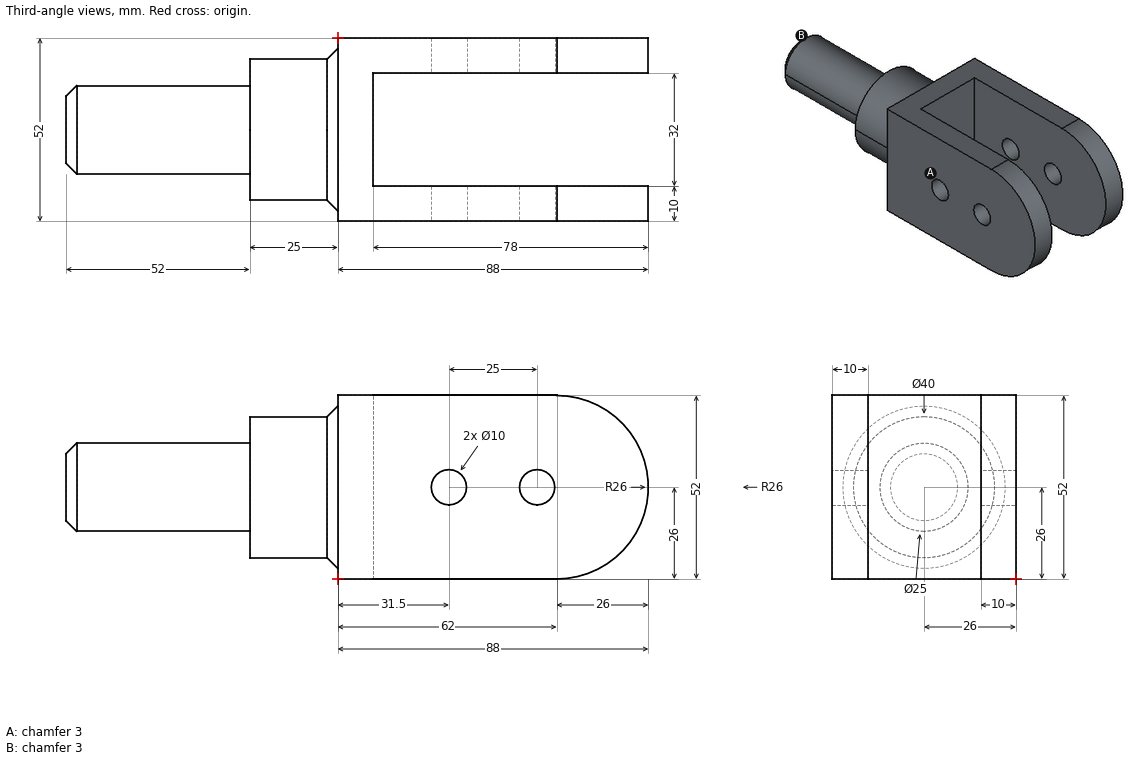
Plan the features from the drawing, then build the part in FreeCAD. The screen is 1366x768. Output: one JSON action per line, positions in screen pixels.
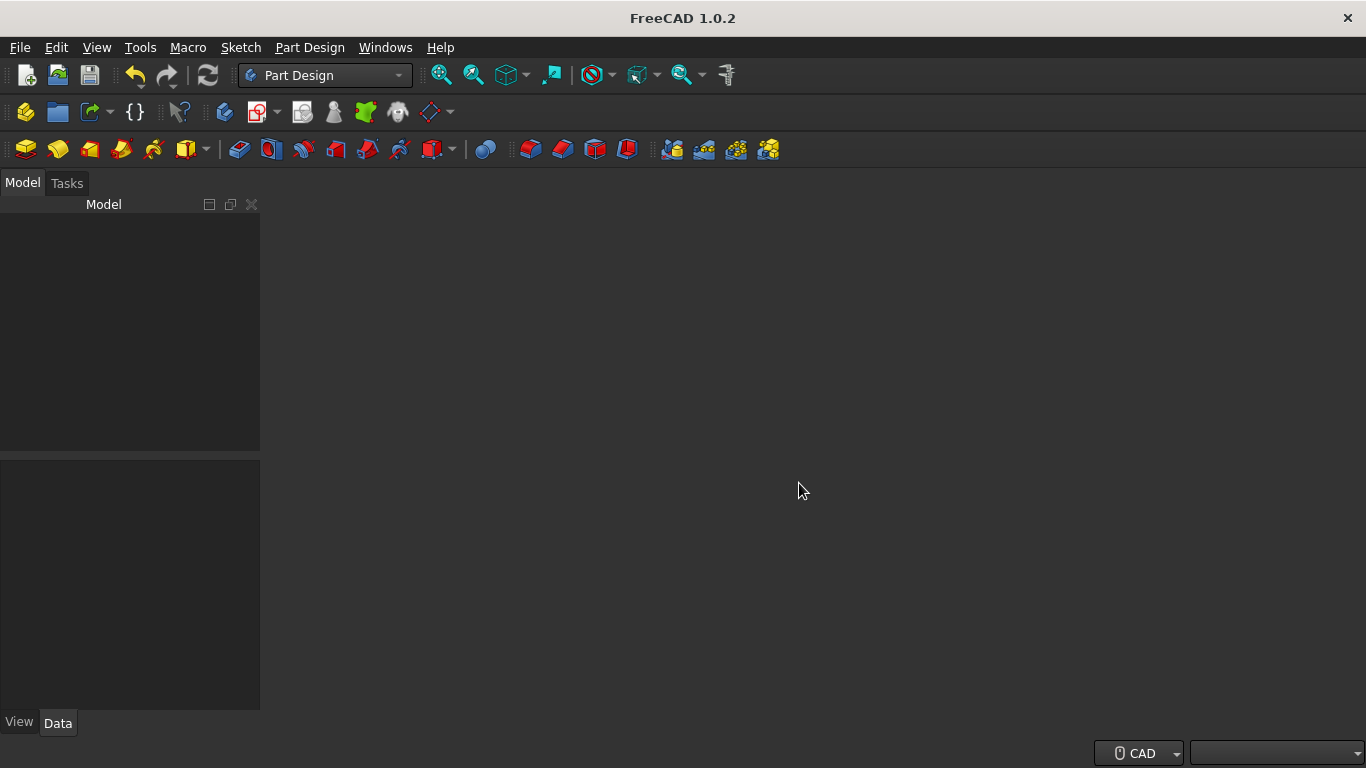
{"action": "left_click", "coordinate": [26, 76]}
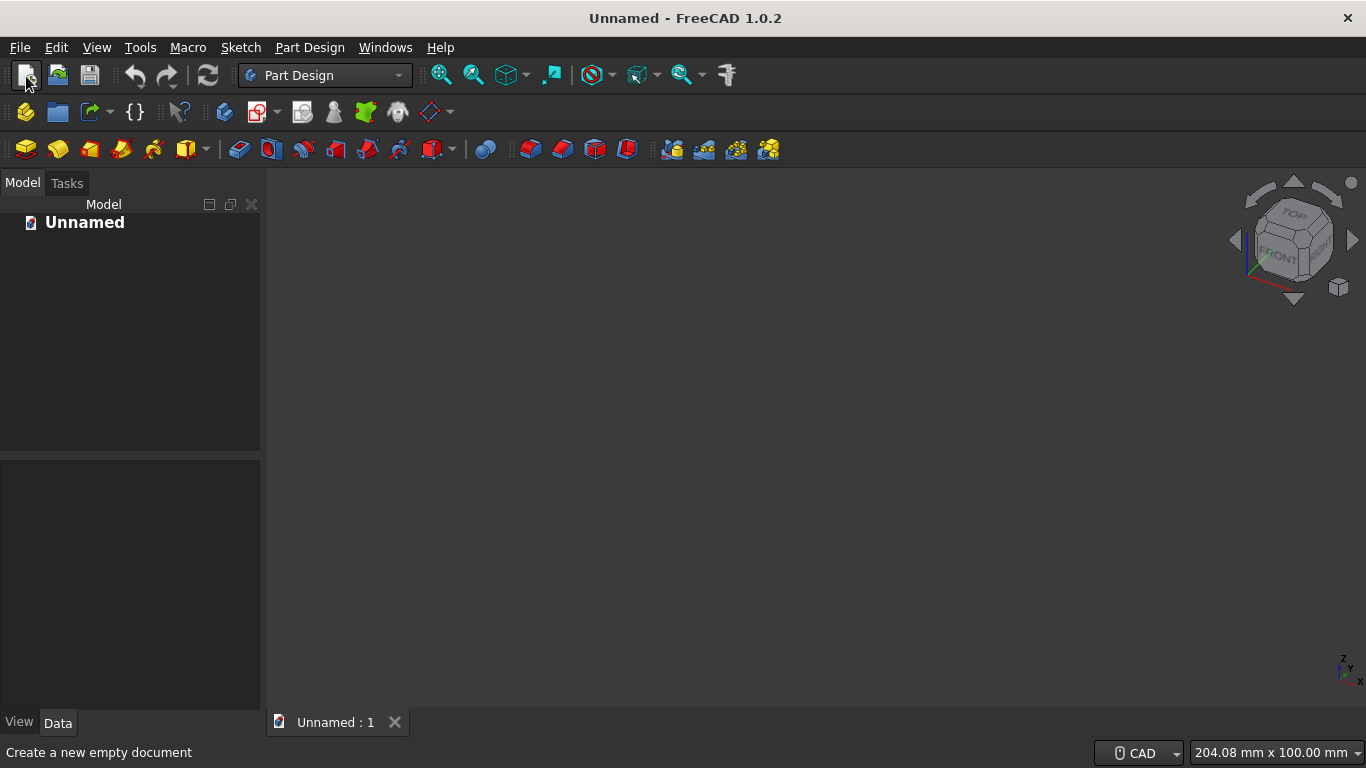
{"action": "left_click", "coordinate": [258, 112]}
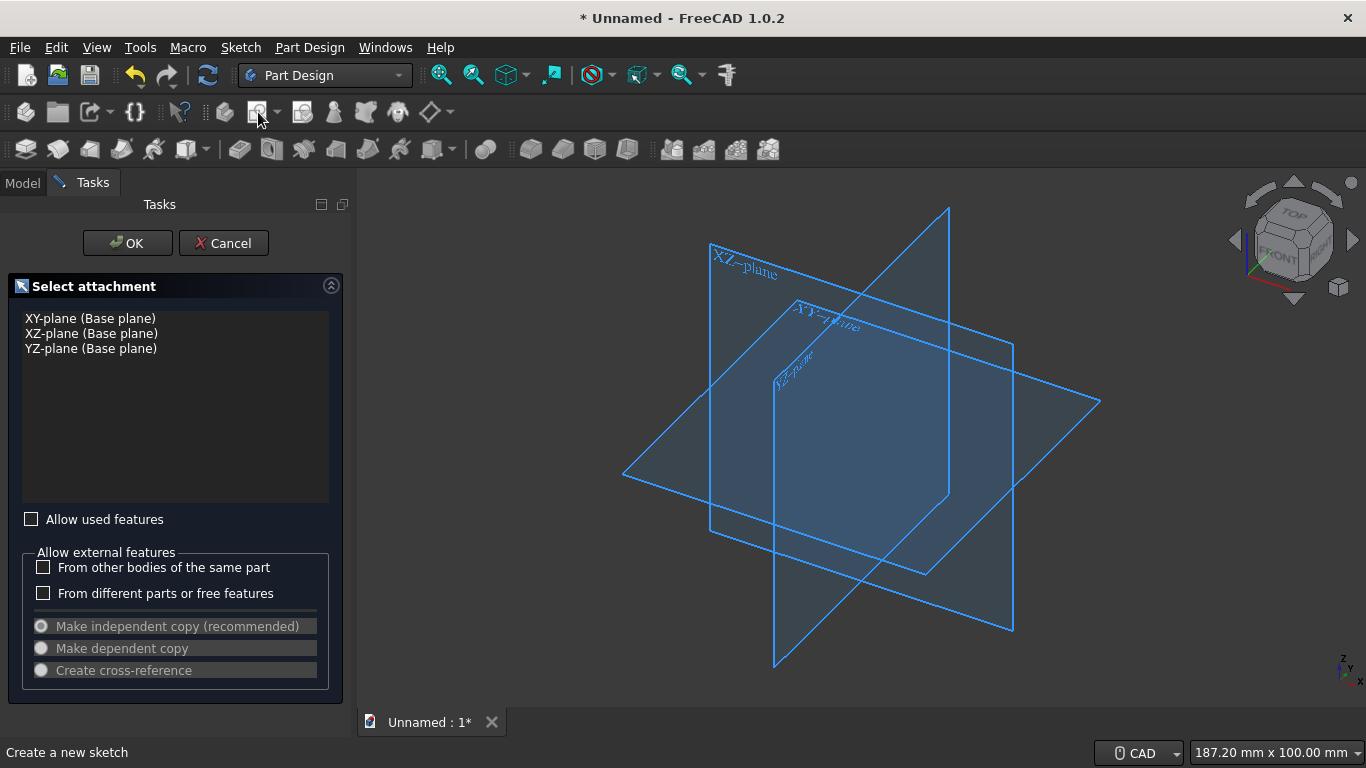
{"action": "left_click", "coordinate": [82, 318]}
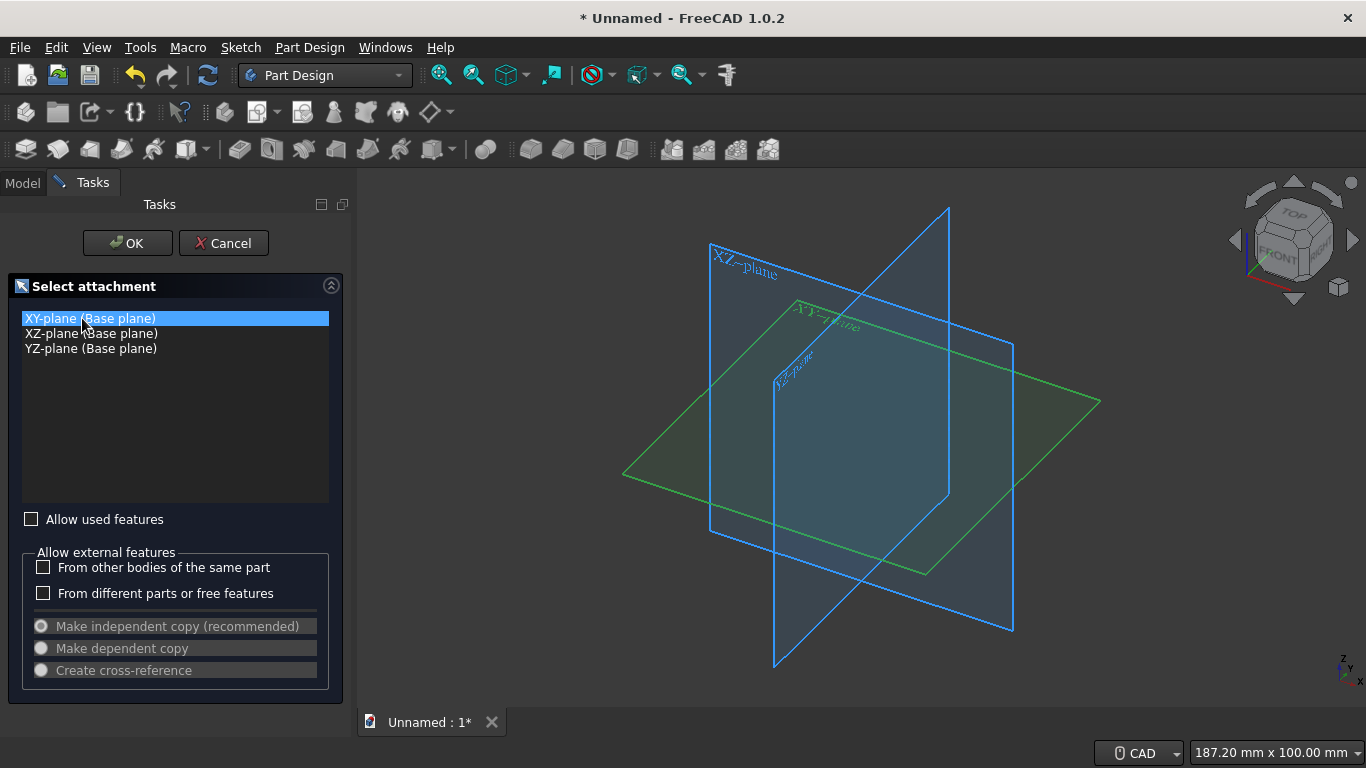
{"action": "left_click", "coordinate": [128, 243]}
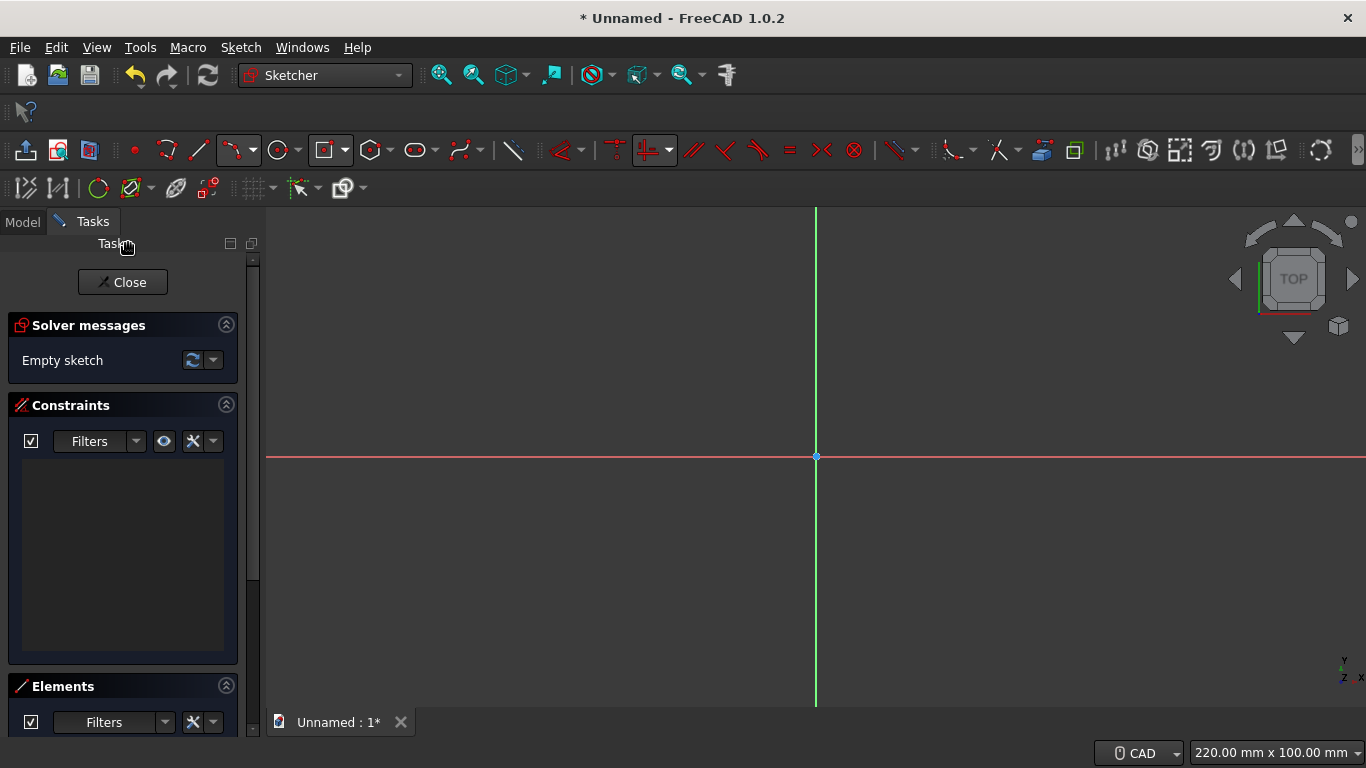
{"action": "scroll", "coordinate": [294, 235], "scroll_direction": "down", "scroll_amount": 1}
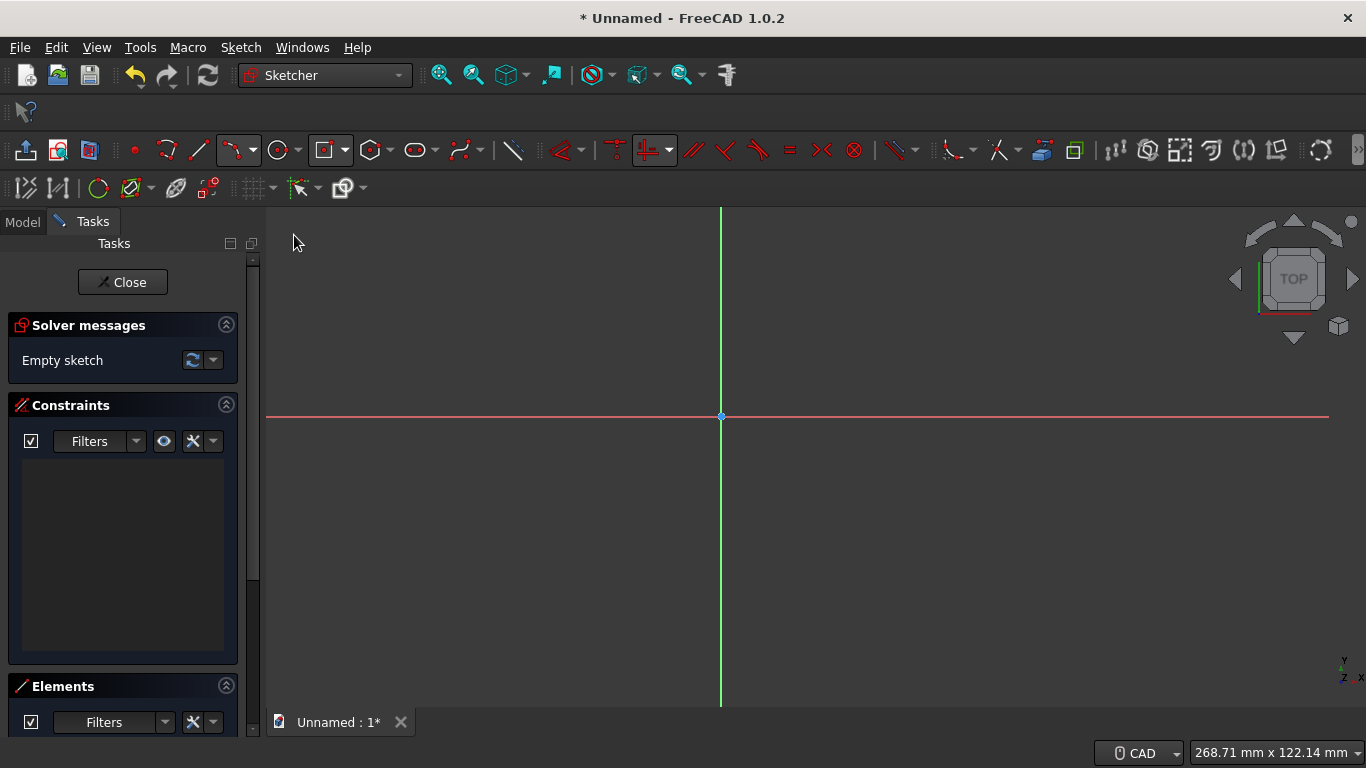
{"action": "scroll", "coordinate": [1201, 658], "scroll_direction": "up", "scroll_amount": 2}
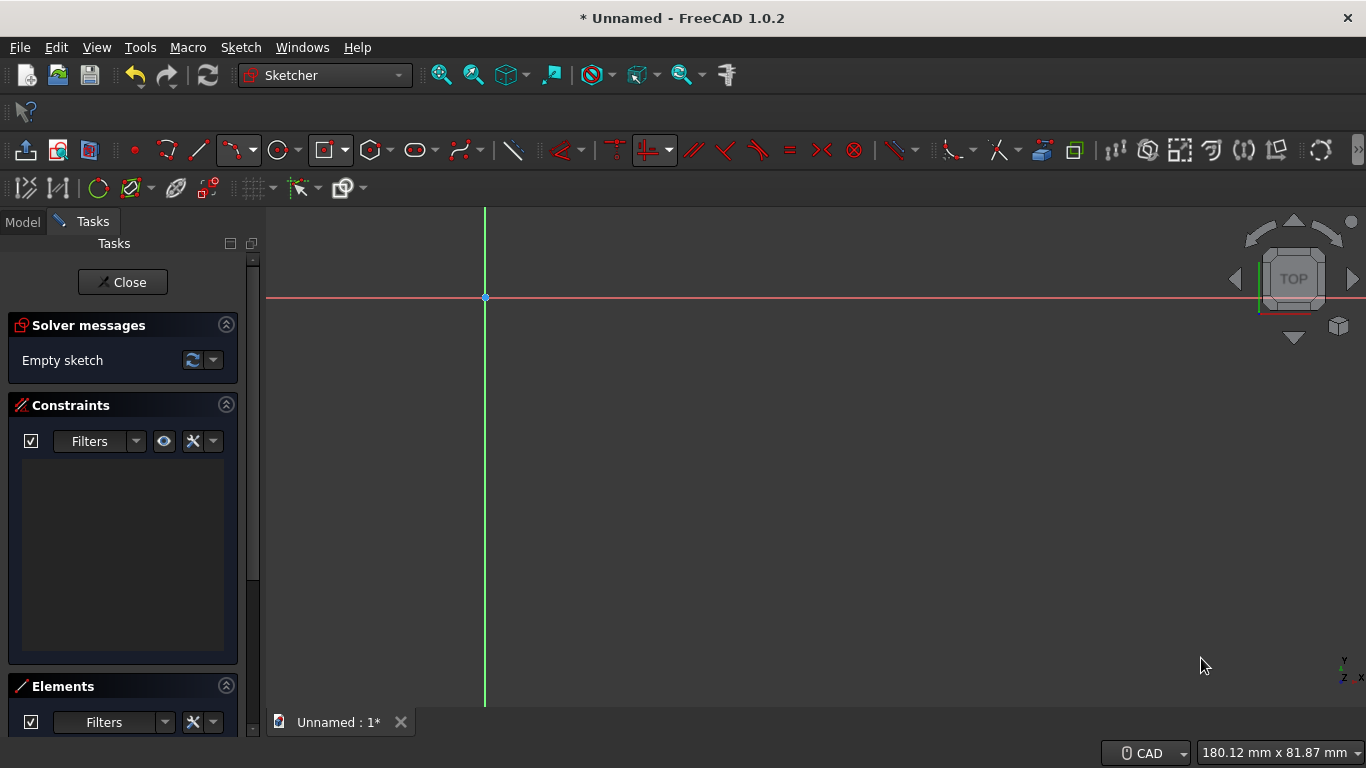
{"action": "left_click", "coordinate": [168, 150]}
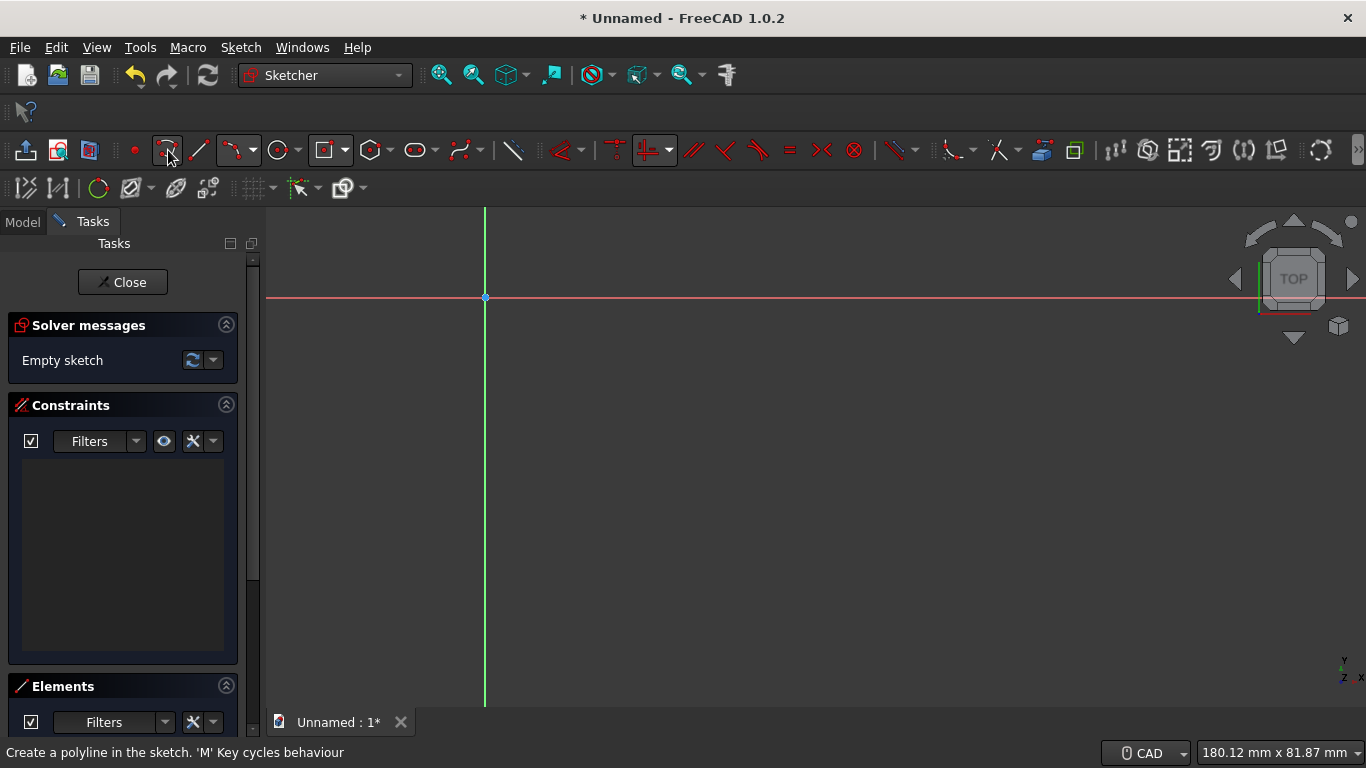
{"action": "left_click", "coordinate": [485, 298]}
{"action": "left_click", "coordinate": [494, 615]}
{"action": "left_click", "coordinate": [1022, 615]}
{"action": "left_click", "coordinate": [1022, 554]}
{"action": "left_click", "coordinate": [546, 554]}
{"action": "left_click", "coordinate": [546, 359]}
{"action": "left_click", "coordinate": [1022, 359]}
{"action": "left_click", "coordinate": [1022, 307]}
{"action": "left_click", "coordinate": [485, 298]}
{"action": "key", "text": "Escape"}
{"action": "key", "text": "Escape"}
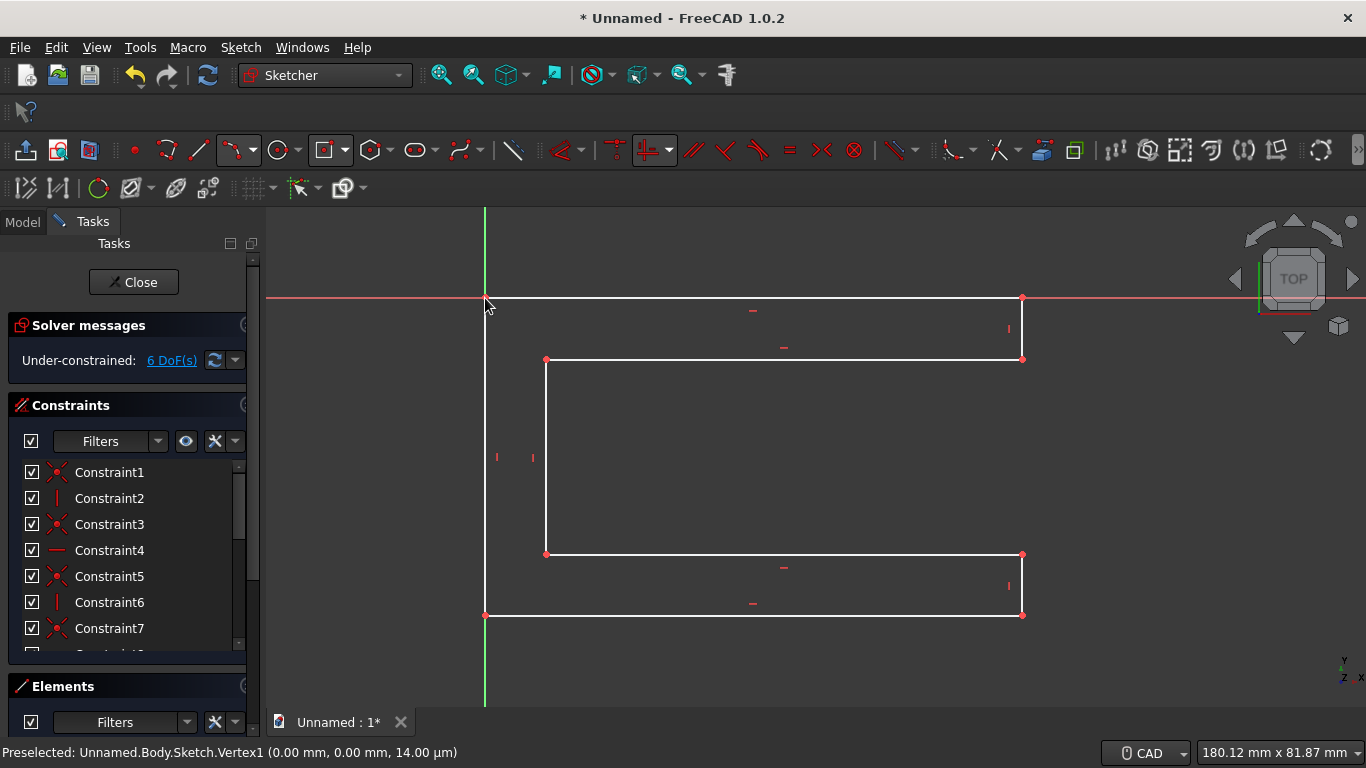
{"action": "left_click", "coordinate": [560, 150]}